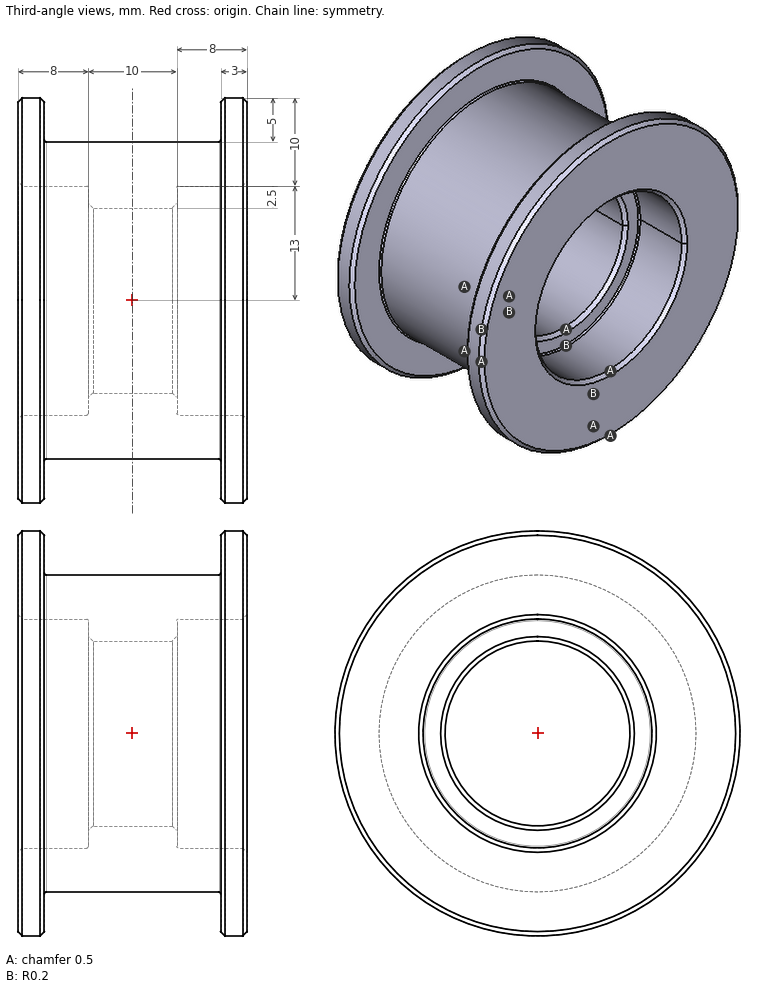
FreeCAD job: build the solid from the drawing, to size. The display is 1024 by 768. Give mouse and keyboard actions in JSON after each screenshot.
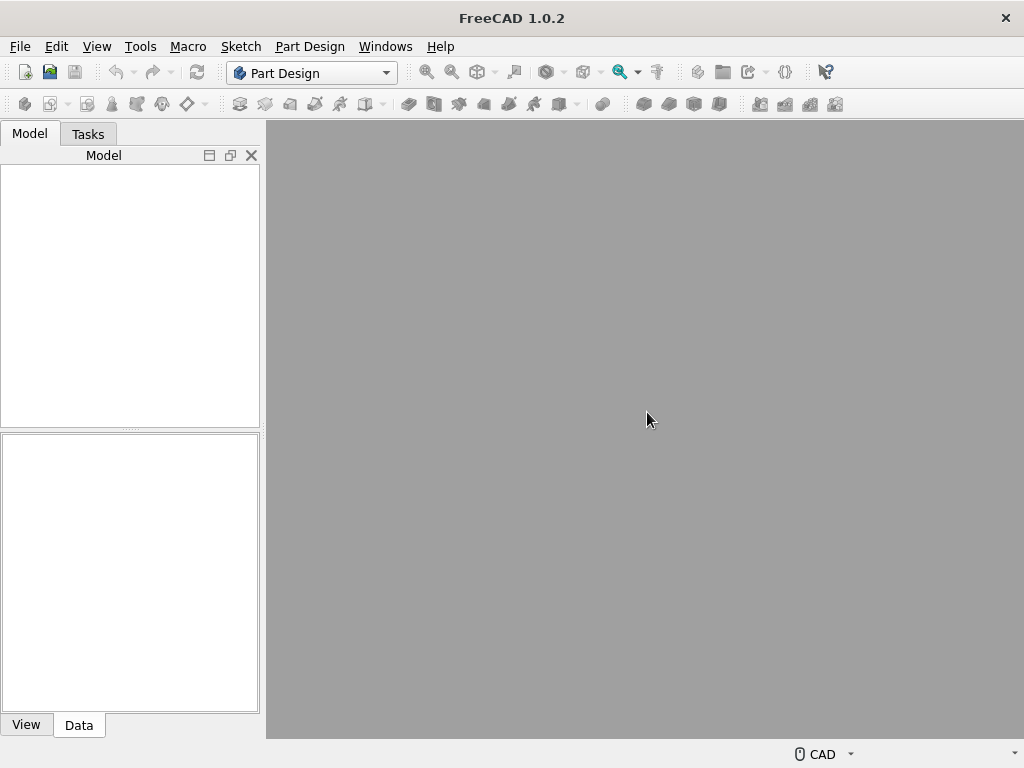
{"action": "left_click", "coordinate": [25, 72]}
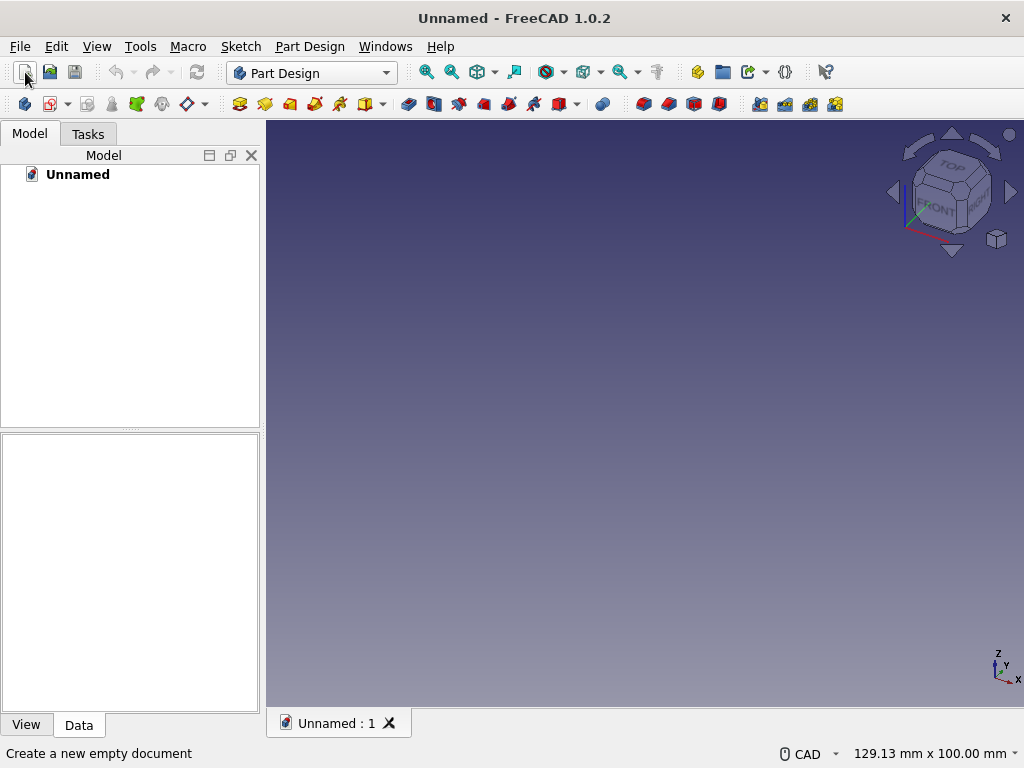
{"action": "left_click", "coordinate": [50, 104]}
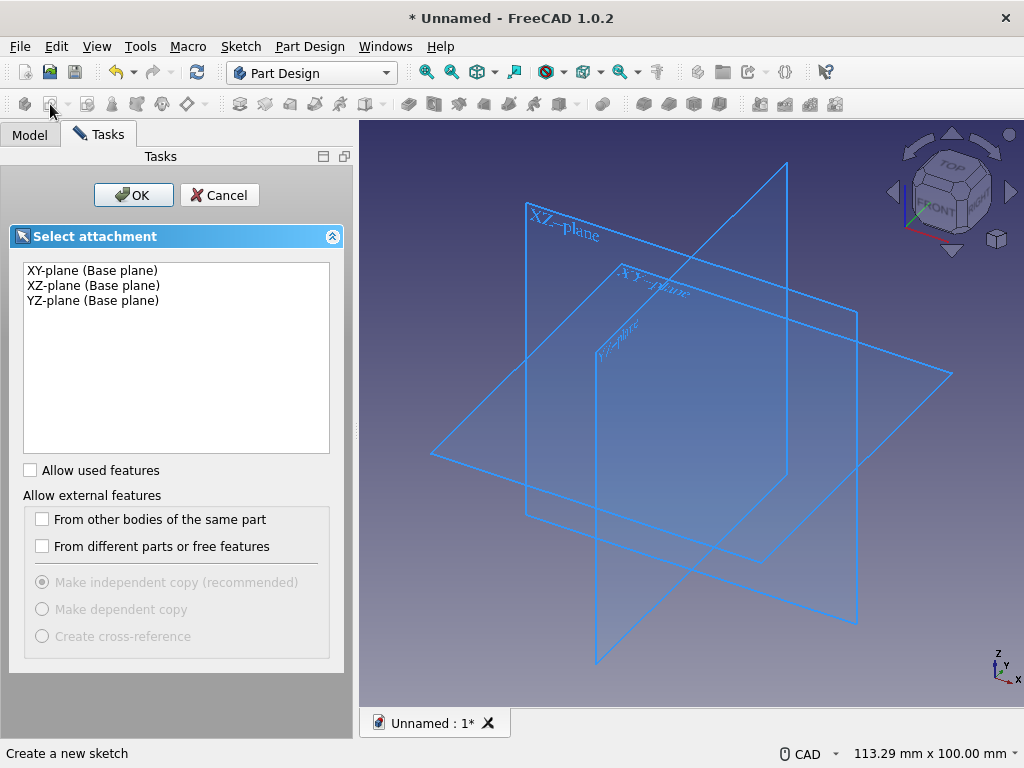
{"action": "left_click", "coordinate": [84, 270]}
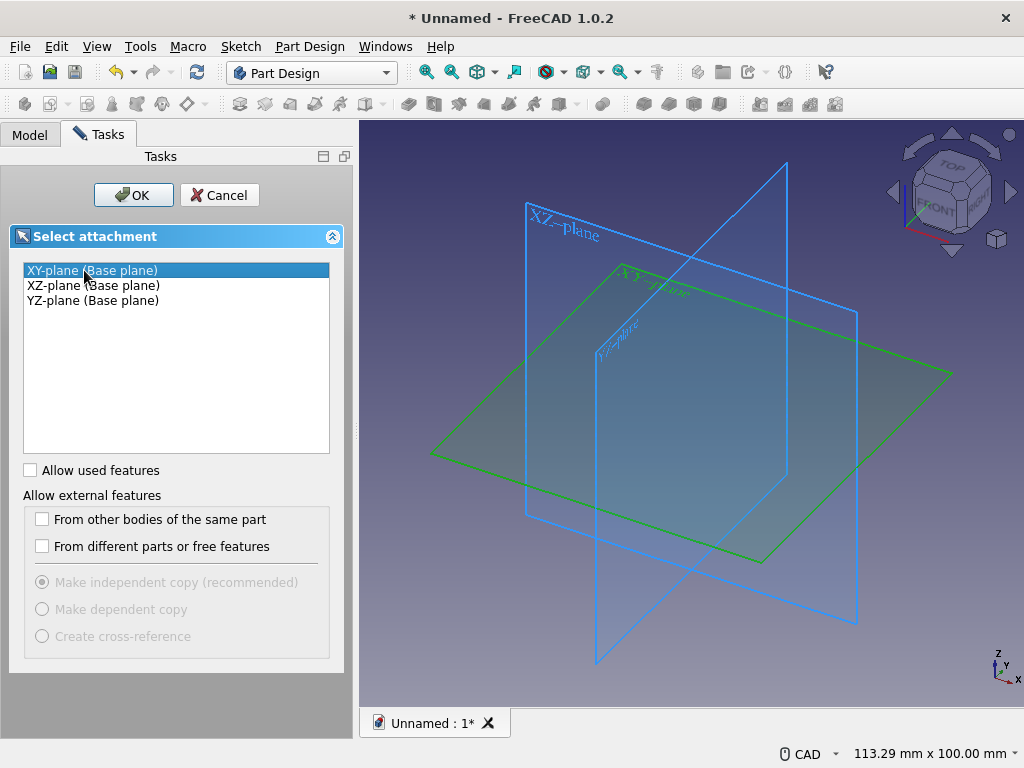
{"action": "left_click", "coordinate": [134, 195]}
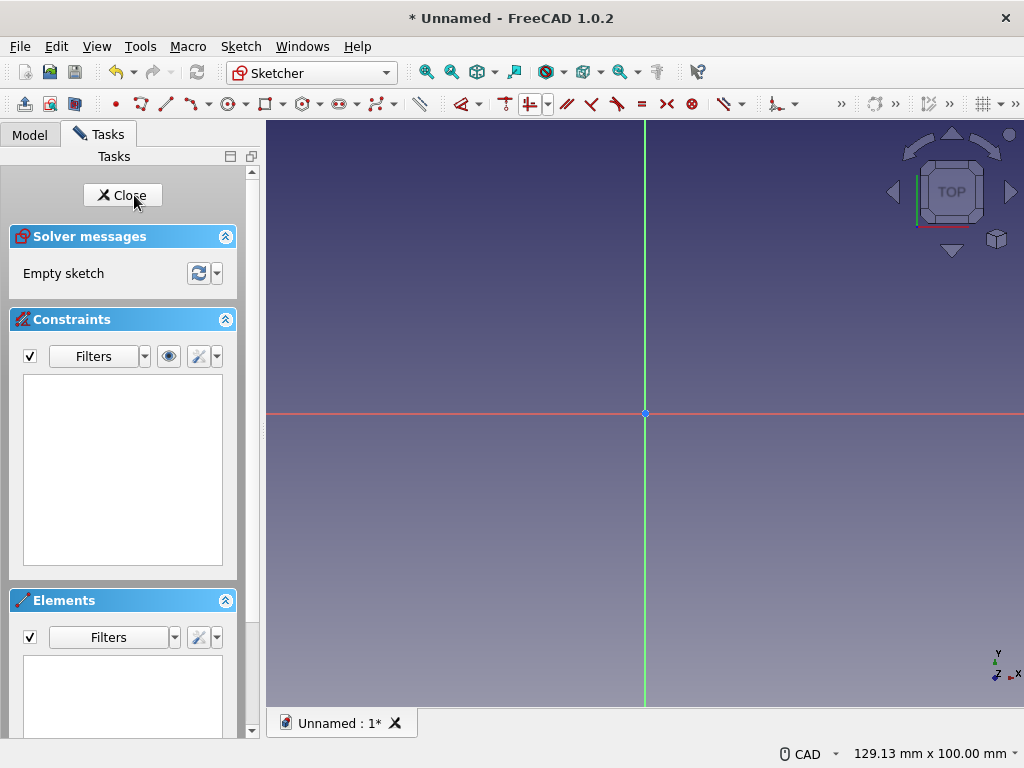
{"action": "scroll", "coordinate": [685, 307], "scroll_direction": "up", "scroll_amount": 5}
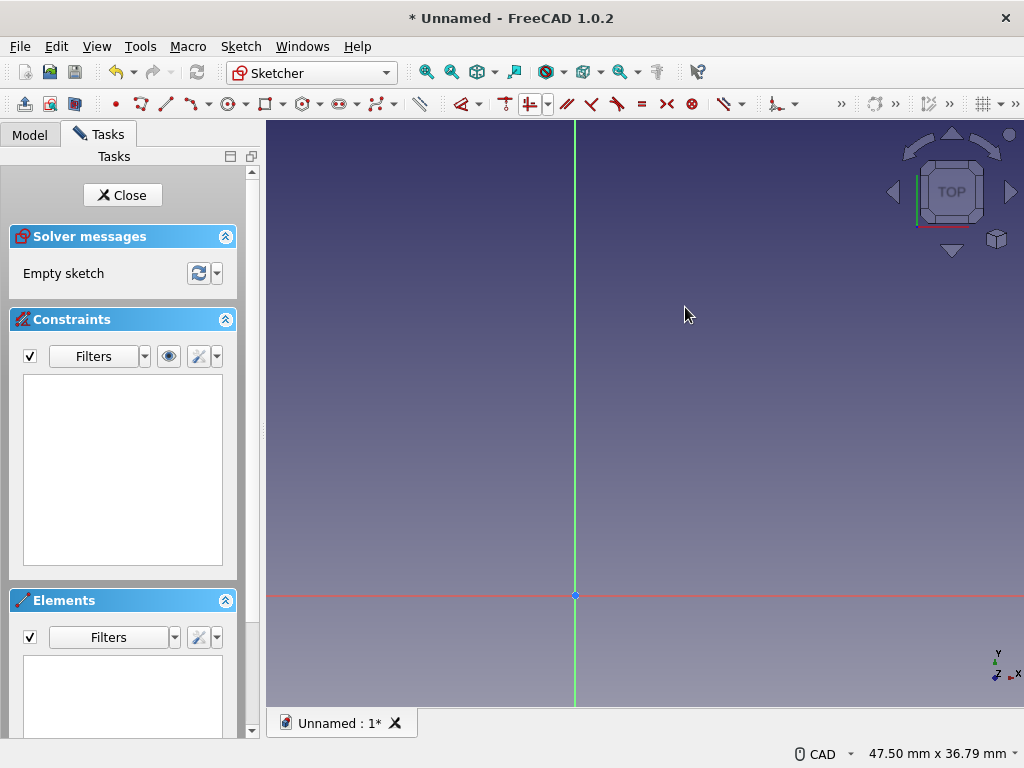
{"action": "left_click", "coordinate": [141, 104]}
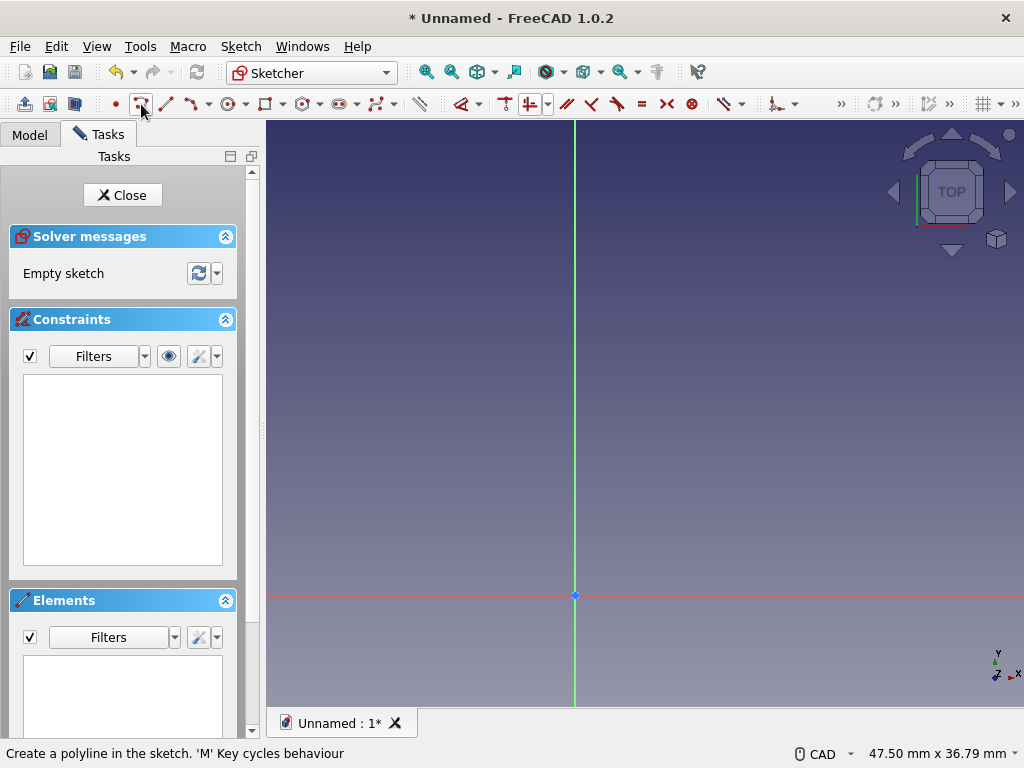
{"action": "left_click", "coordinate": [496, 428]}
{"action": "left_click", "coordinate": [655, 428]}
{"action": "left_click", "coordinate": [655, 389]}
{"action": "left_click", "coordinate": [783, 389]}
{"action": "left_click", "coordinate": [783, 229]}
{"action": "left_click", "coordinate": [735, 229]}
{"action": "left_click", "coordinate": [735, 309]}
{"action": "left_click", "coordinate": [416, 309]}
{"action": "left_click", "coordinate": [416, 229]}
{"action": "left_click", "coordinate": [368, 229]}
{"action": "left_click", "coordinate": [368, 389]}
{"action": "left_click", "coordinate": [496, 389]}
{"action": "left_click", "coordinate": [496, 429]}
{"action": "key", "text": "Escape"}
{"action": "key", "text": "Escape"}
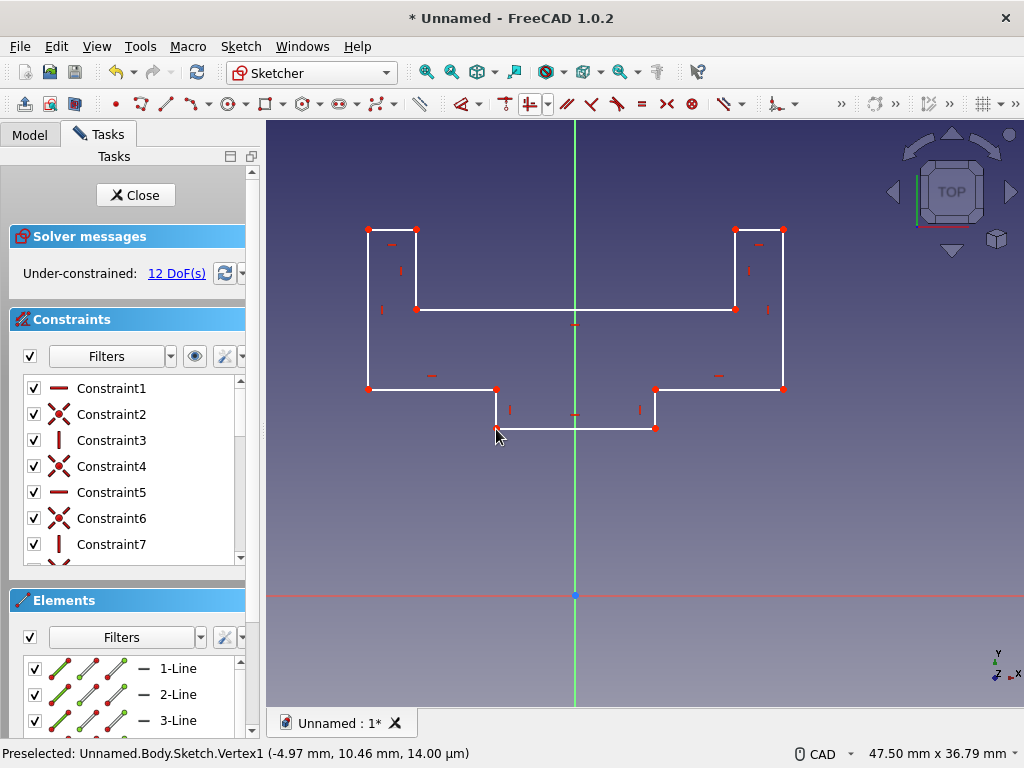
{"action": "left_click", "coordinate": [735, 230]}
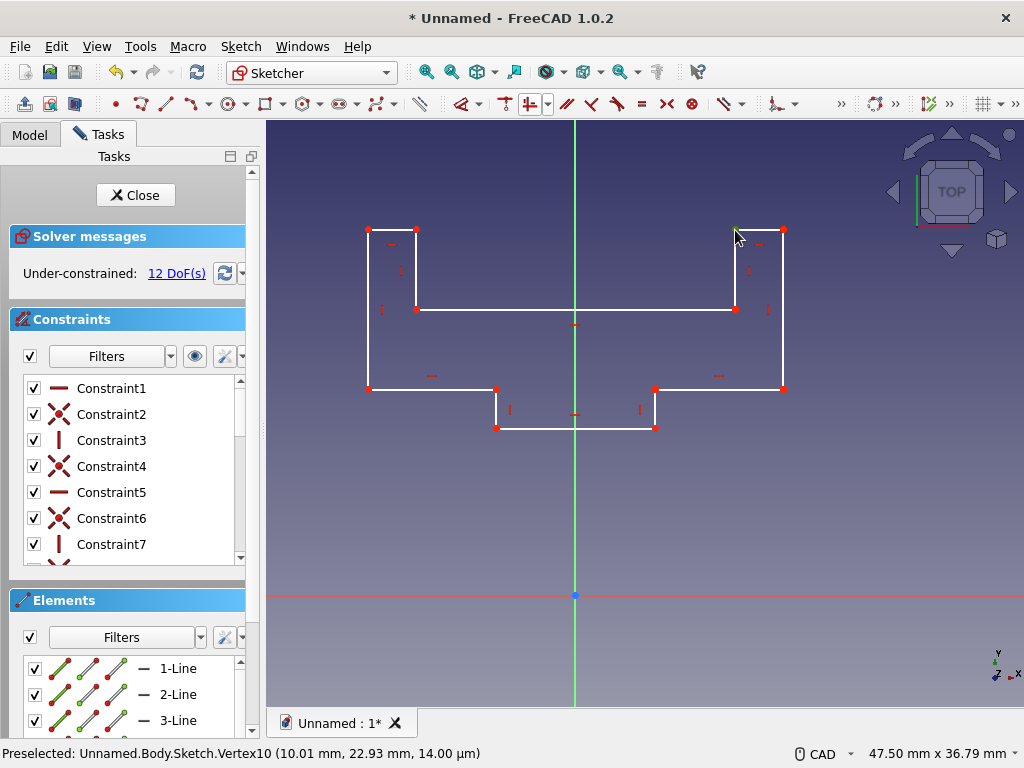
{"action": "left_click", "coordinate": [416, 230]}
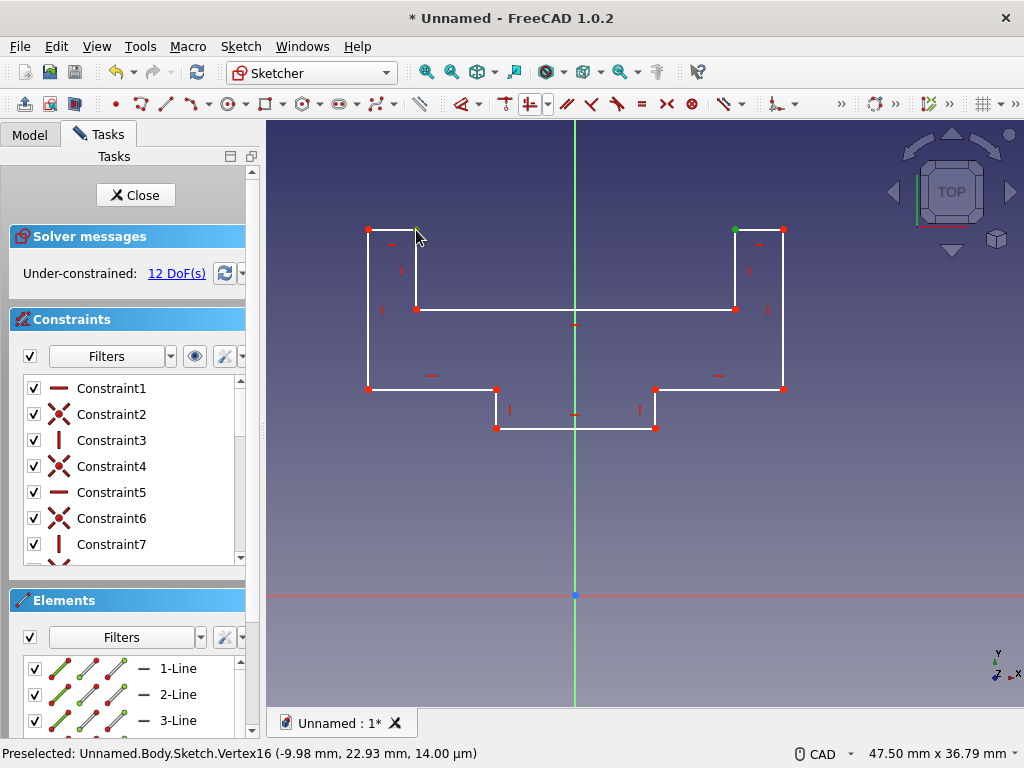
{"action": "left_click", "coordinate": [575, 641]}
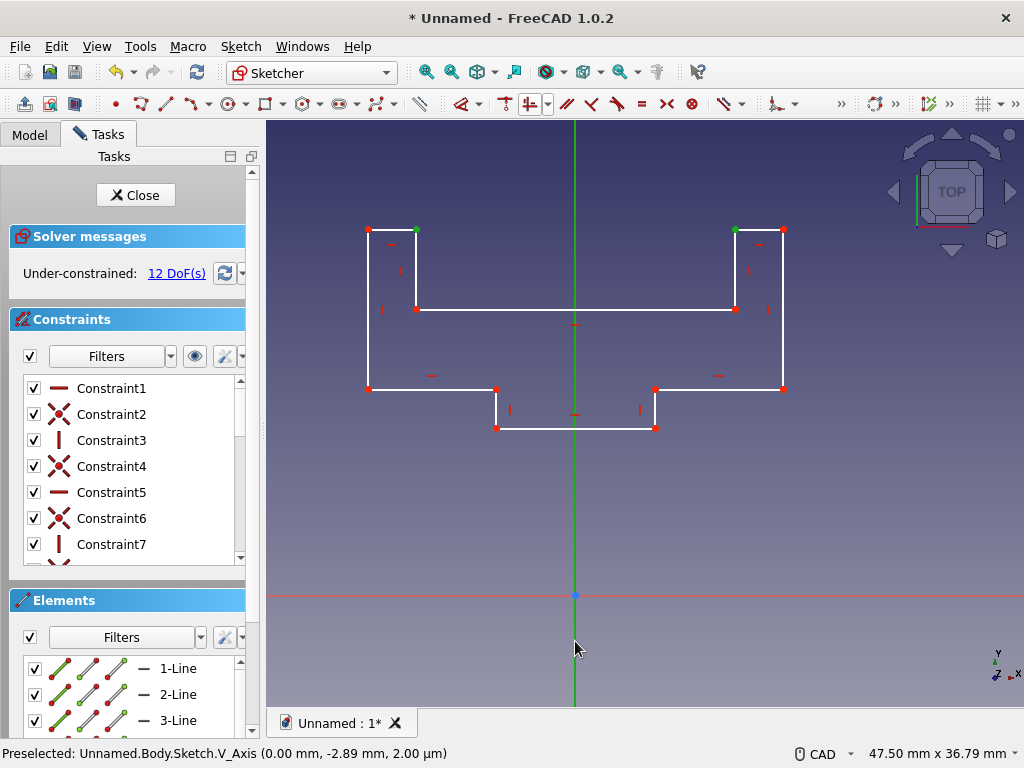
{"action": "left_click", "coordinate": [667, 104]}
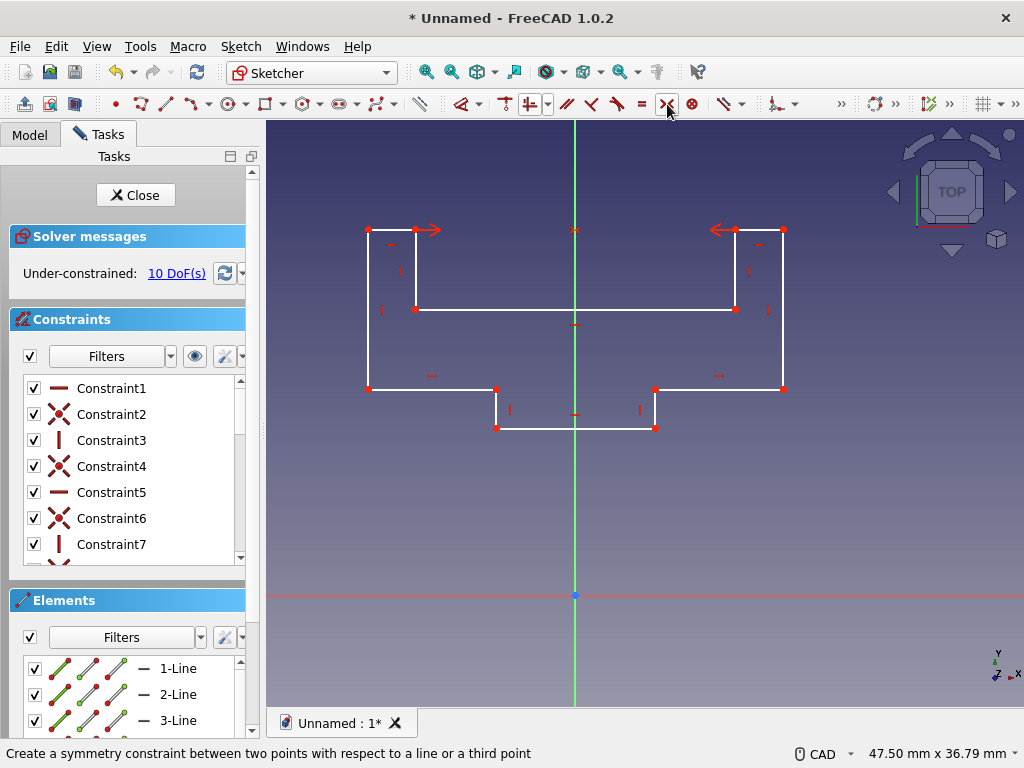
{"action": "left_click", "coordinate": [783, 390]}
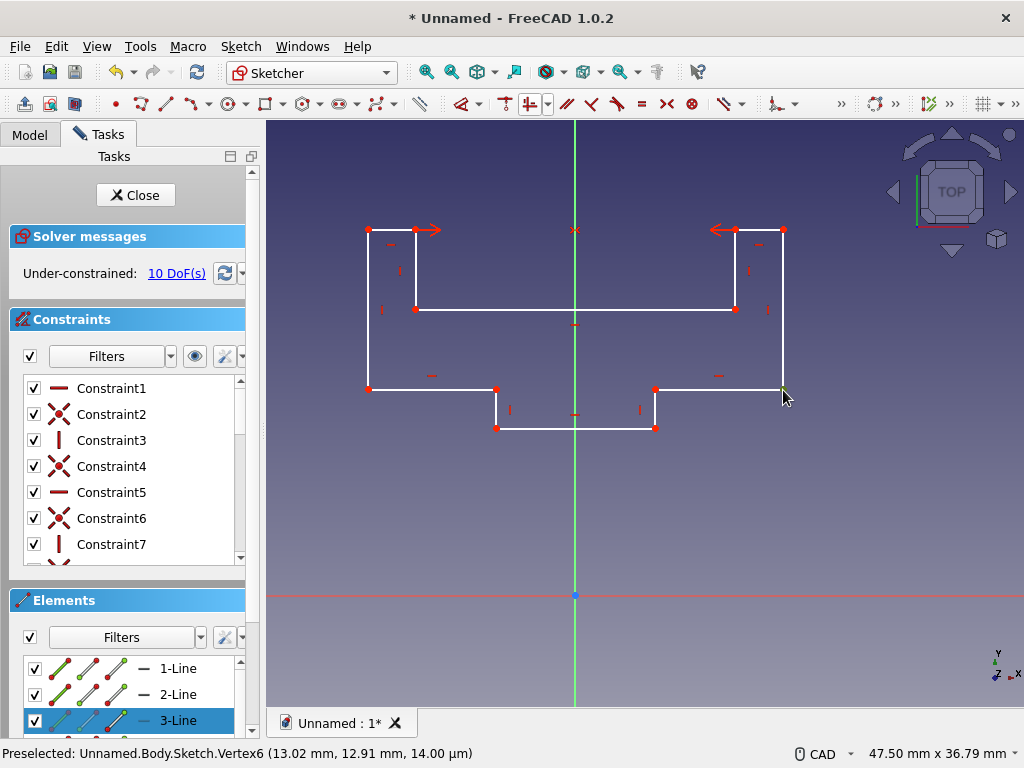
{"action": "left_click", "coordinate": [368, 390]}